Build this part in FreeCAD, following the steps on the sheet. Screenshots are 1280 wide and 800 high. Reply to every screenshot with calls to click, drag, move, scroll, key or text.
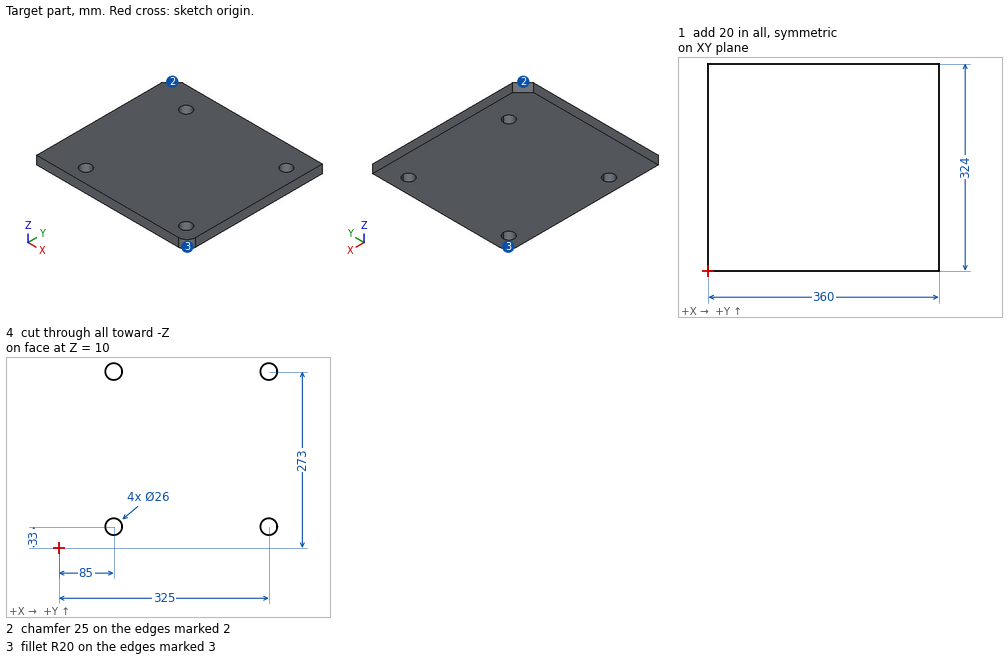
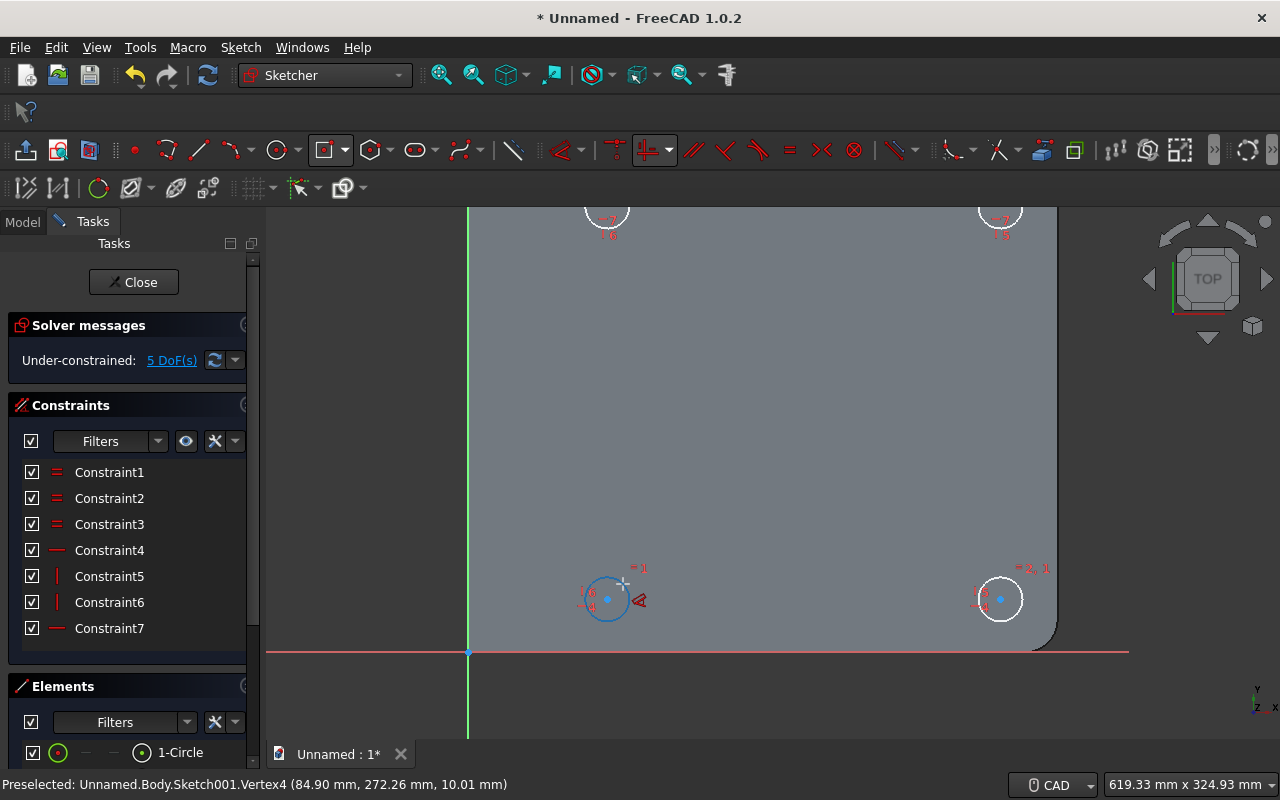
click(623, 584)
click(646, 562)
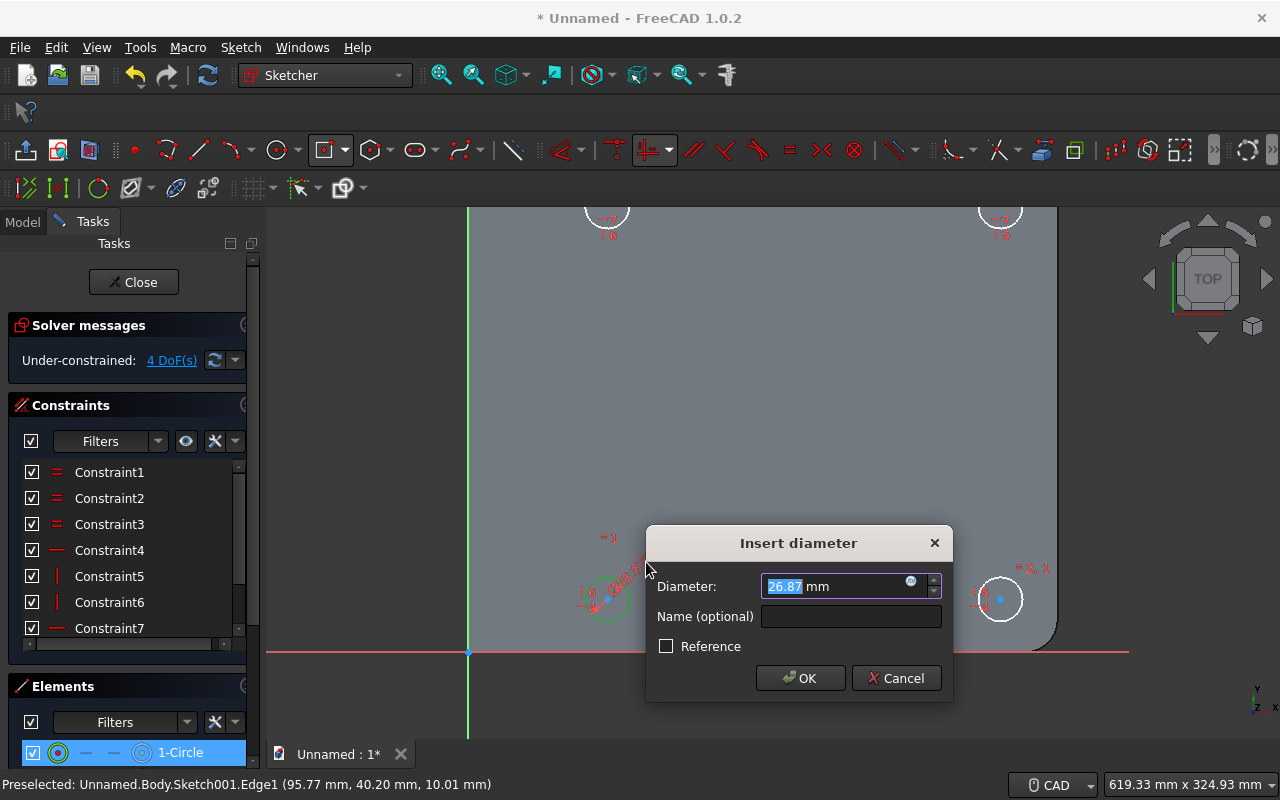
text(26)
key(Return)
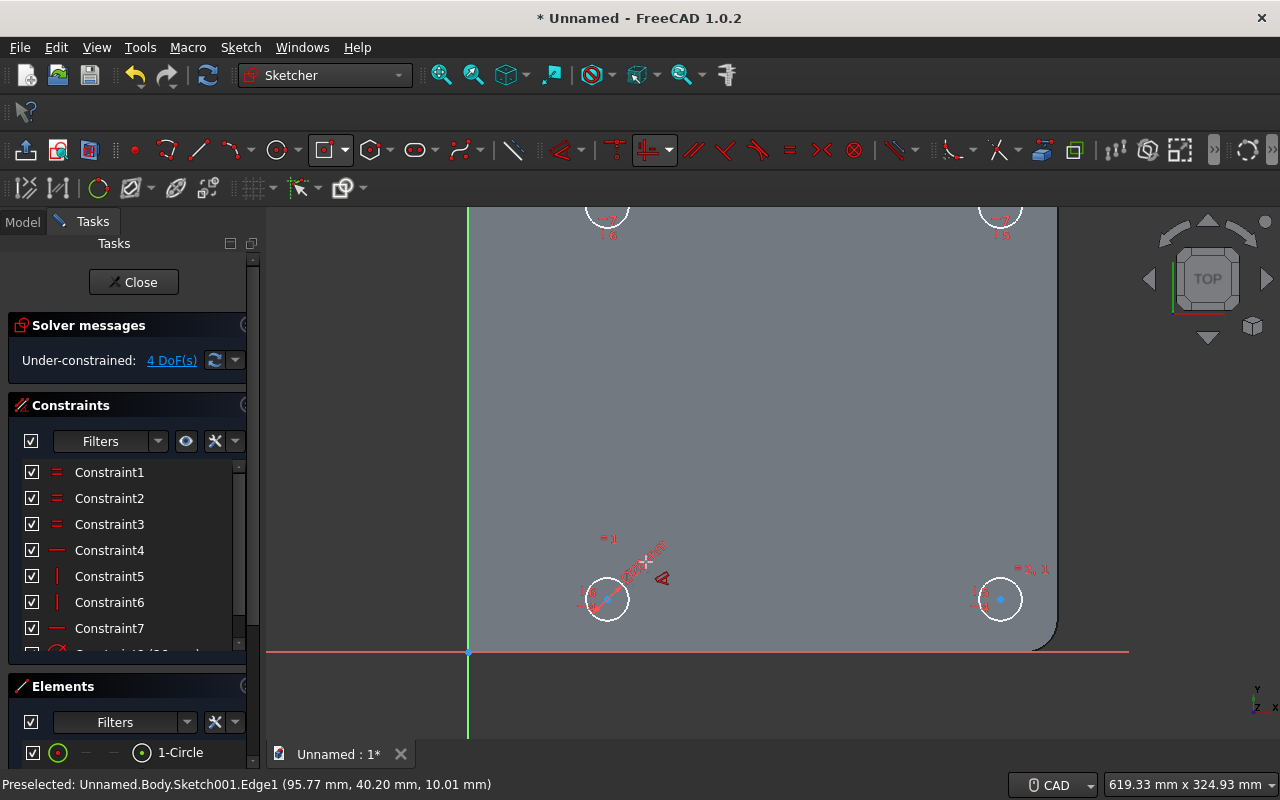
click(607, 599)
click(538, 686)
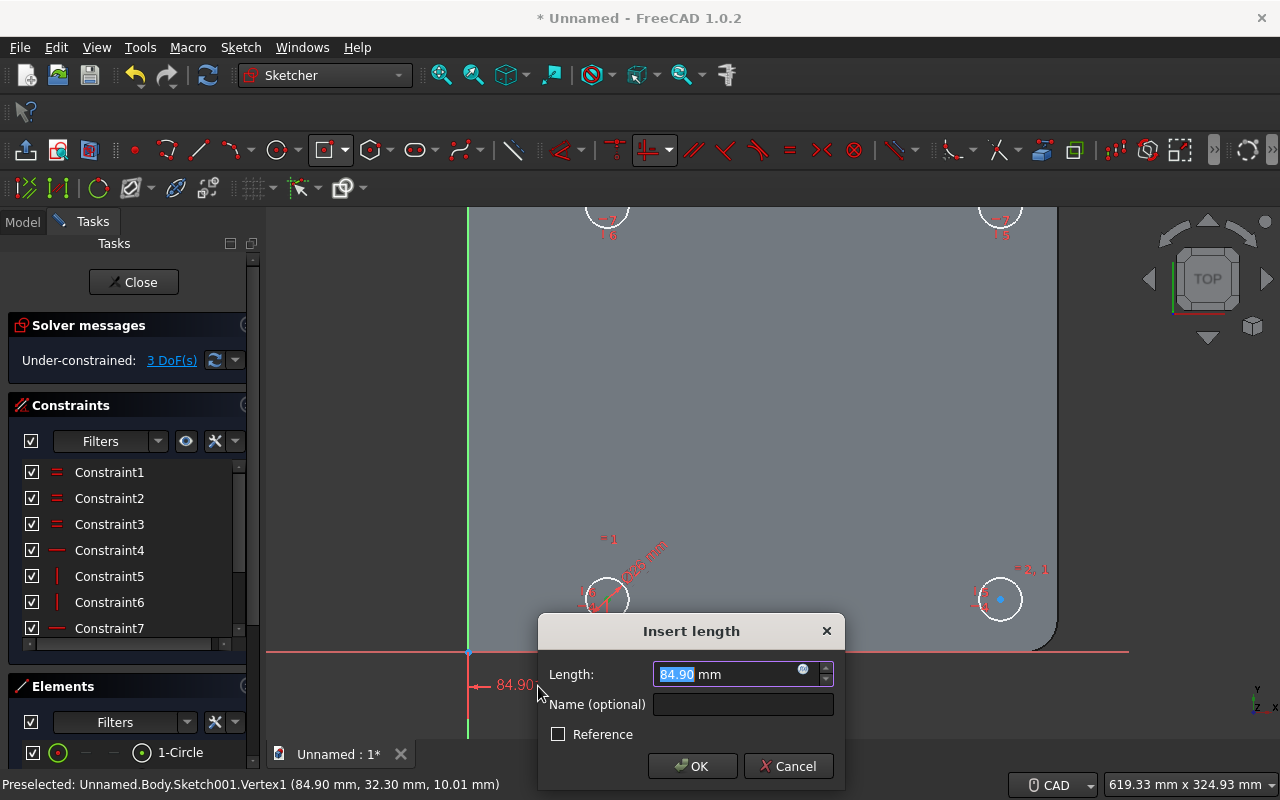
text(85)
key(Return)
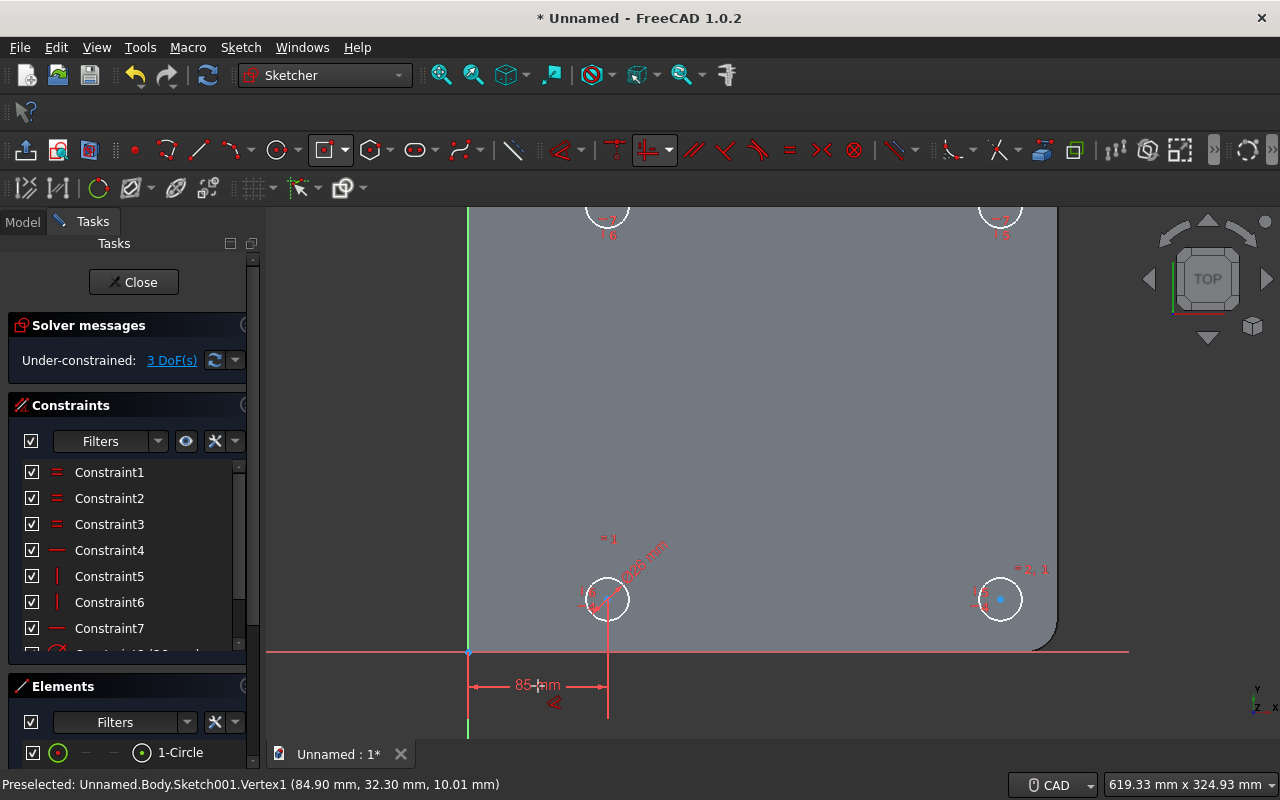
click(608, 599)
click(434, 626)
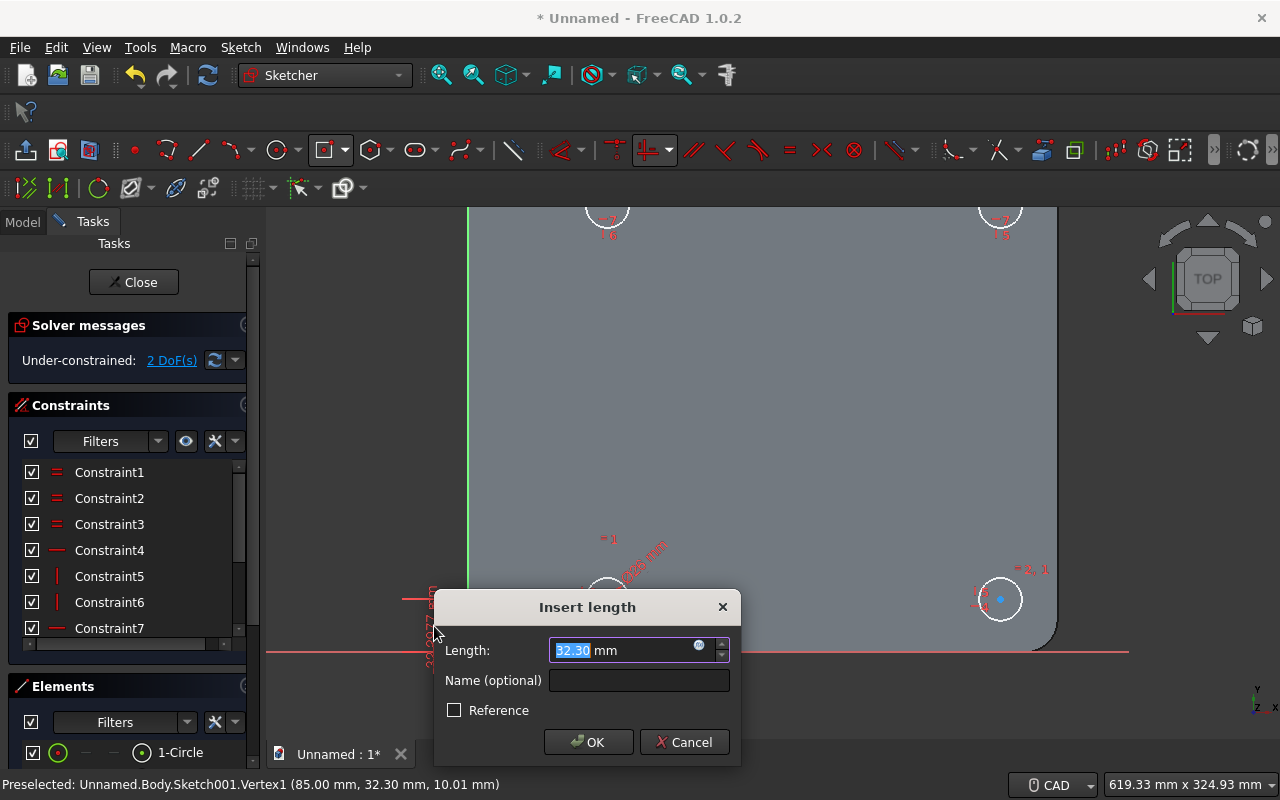
text(33)
key(Return)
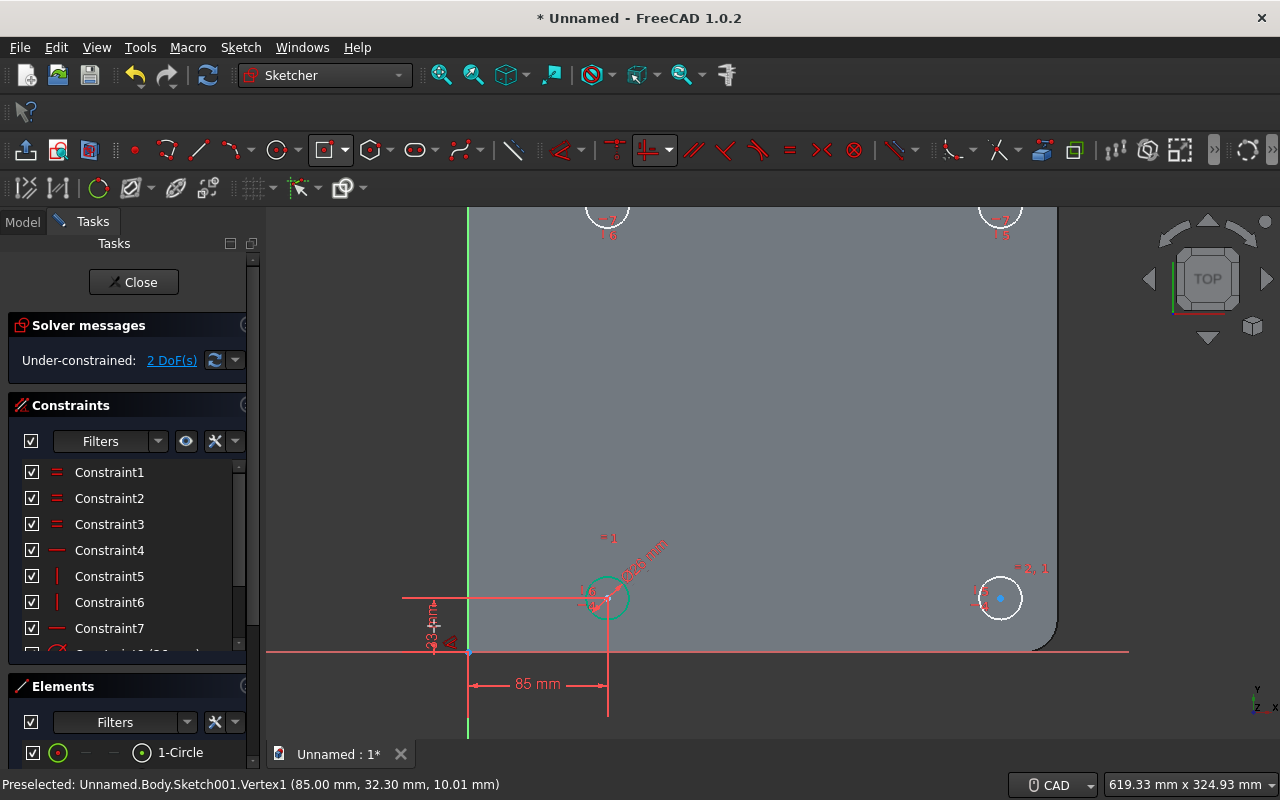
click(1001, 598)
click(734, 686)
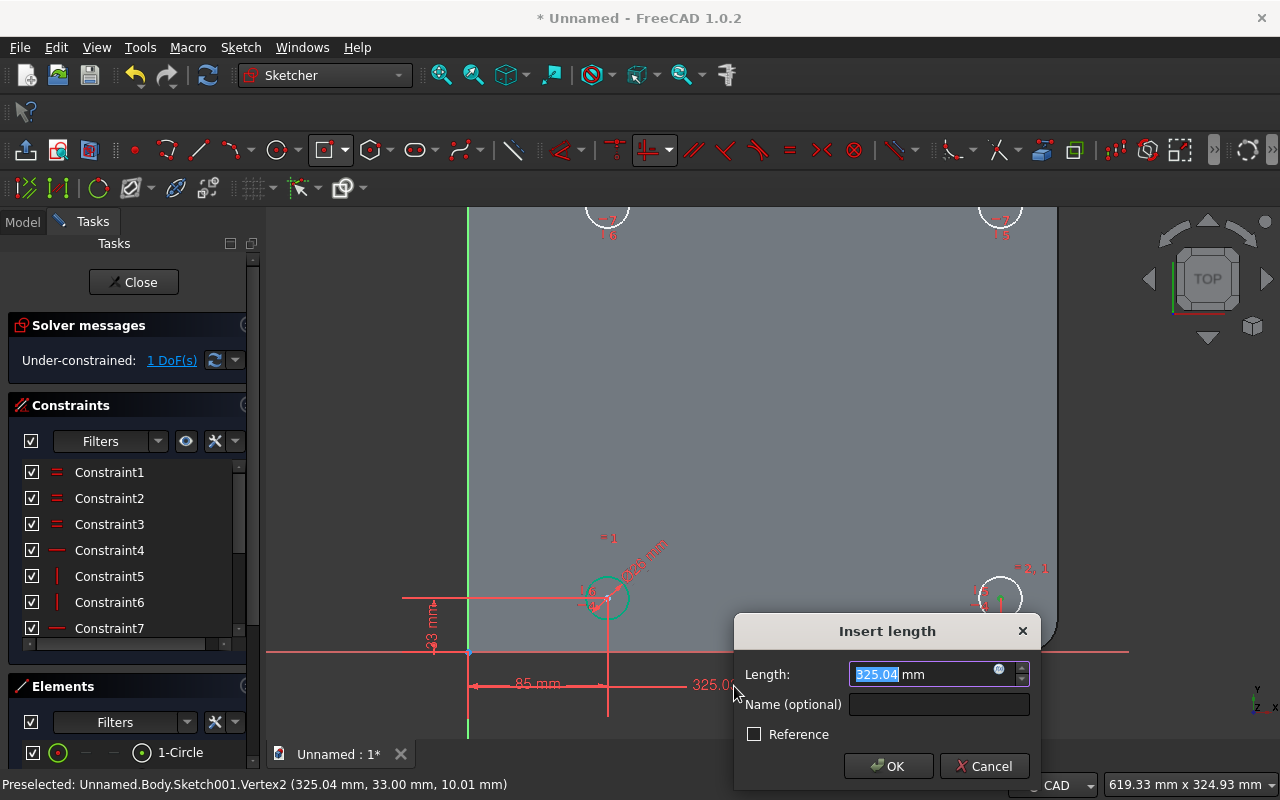
text(325)
key(Return)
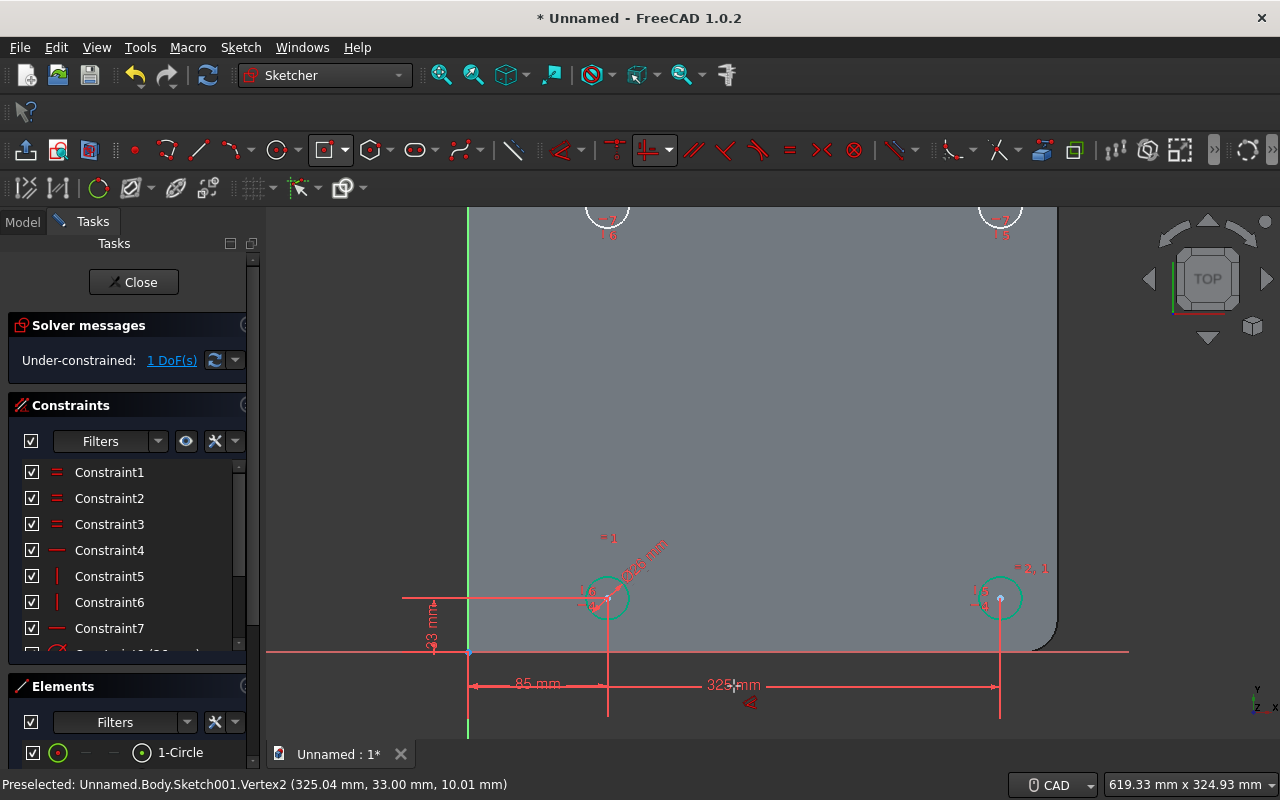
scroll(622, 585, down, 2)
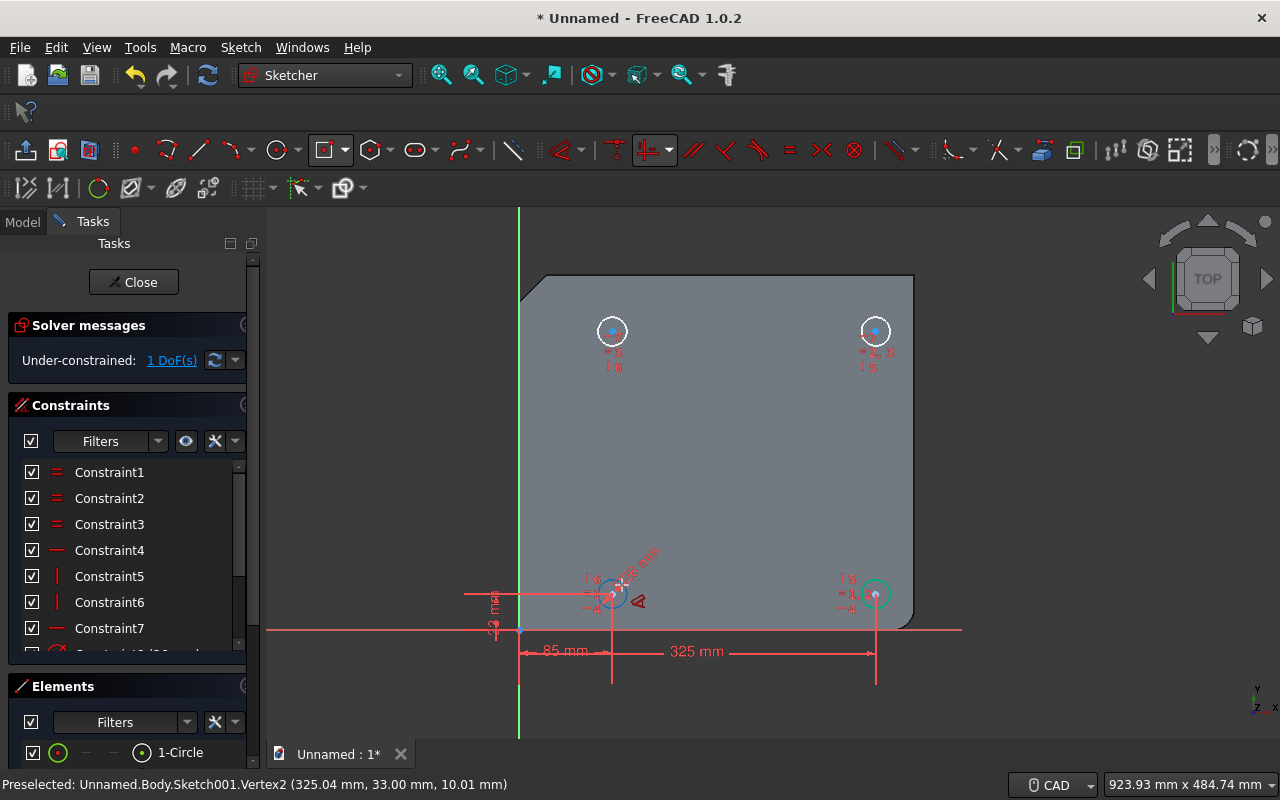
click(876, 332)
click(485, 481)